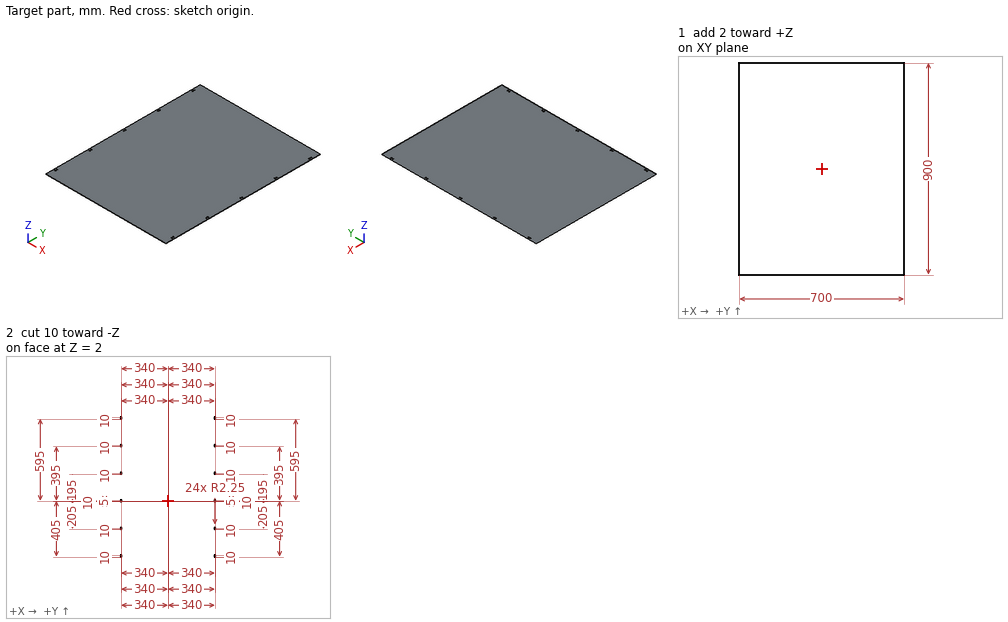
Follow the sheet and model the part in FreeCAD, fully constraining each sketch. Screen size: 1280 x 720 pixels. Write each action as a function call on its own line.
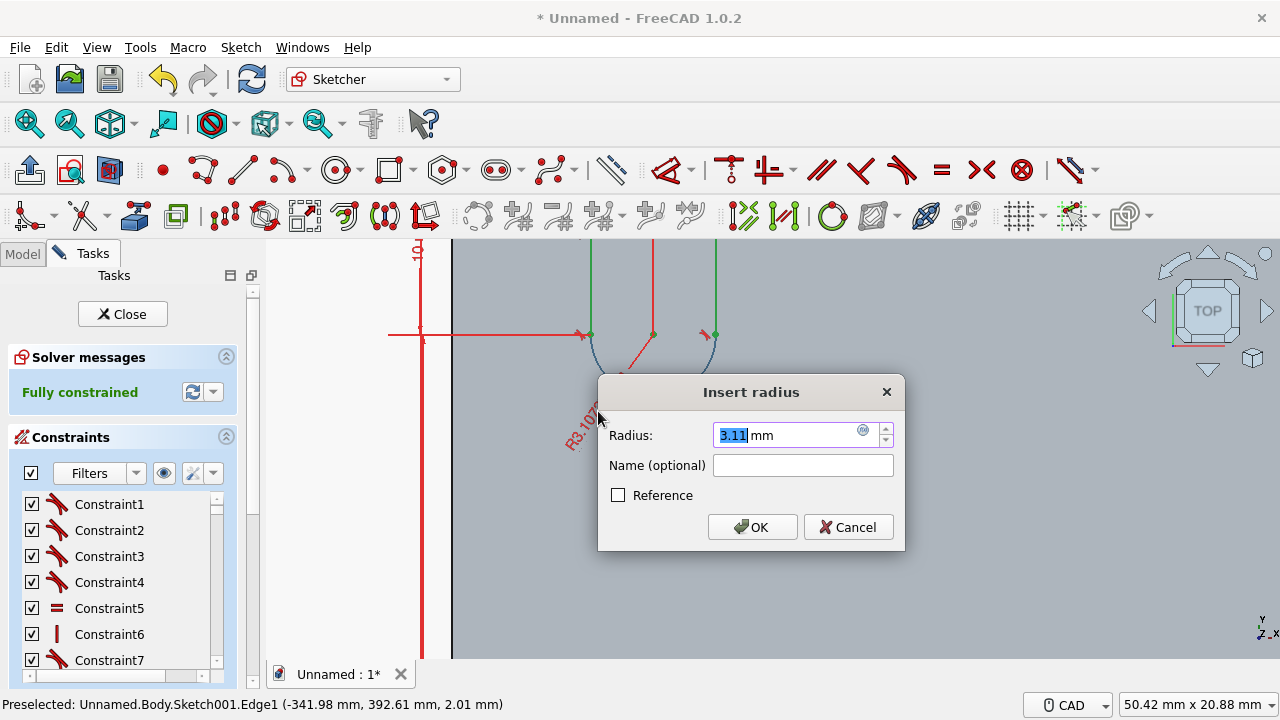
text(2.25)
key(Return)
key(Escape)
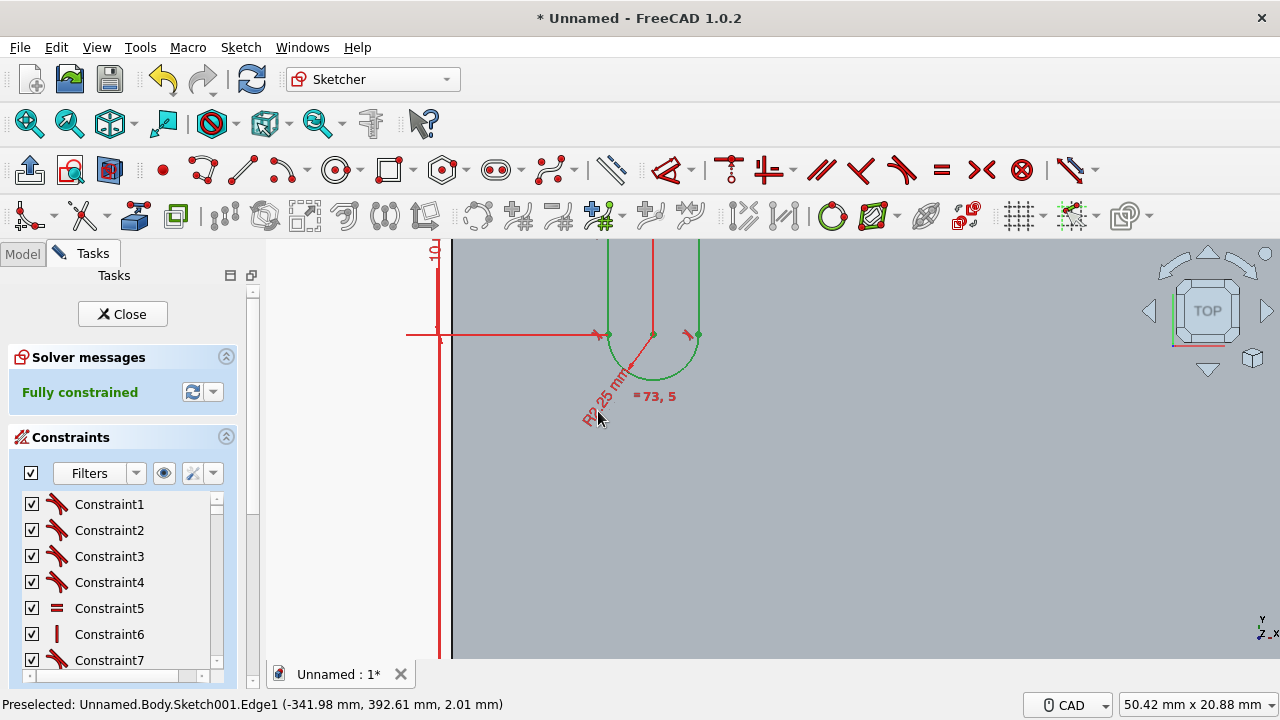
click(123, 314)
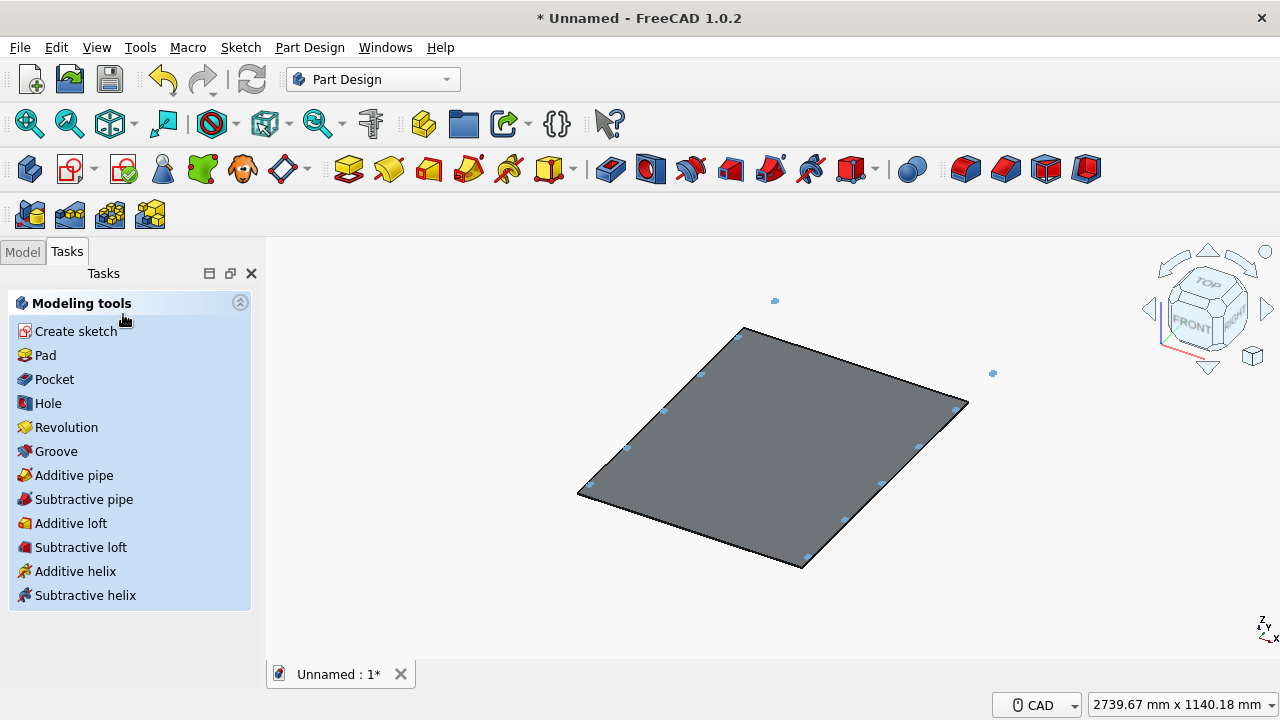
click(612, 170)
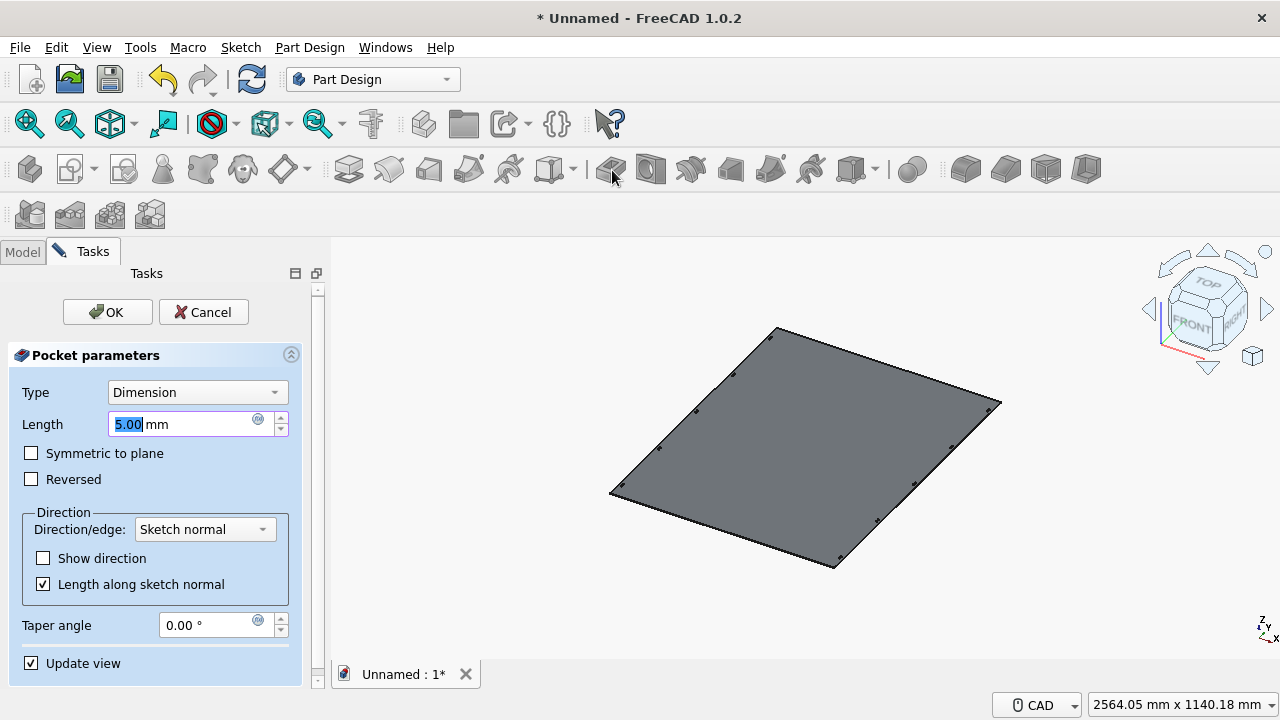
text(10)
key(Tab)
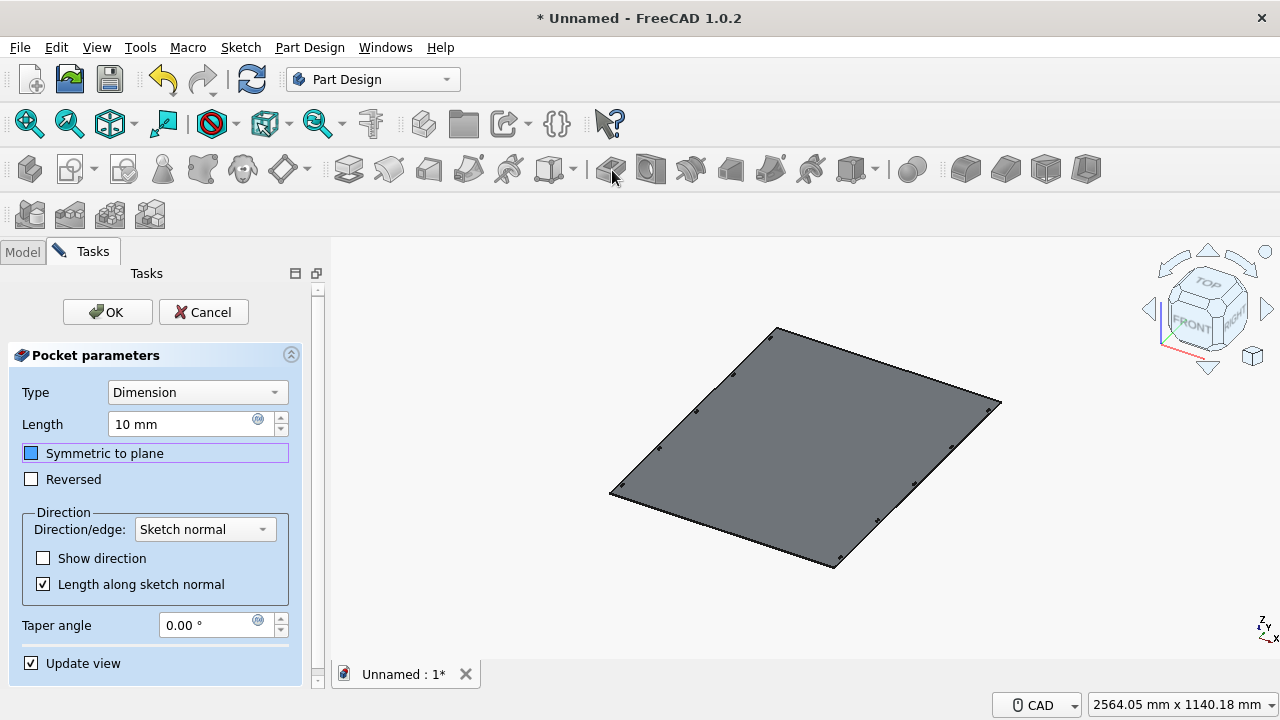
click(108, 312)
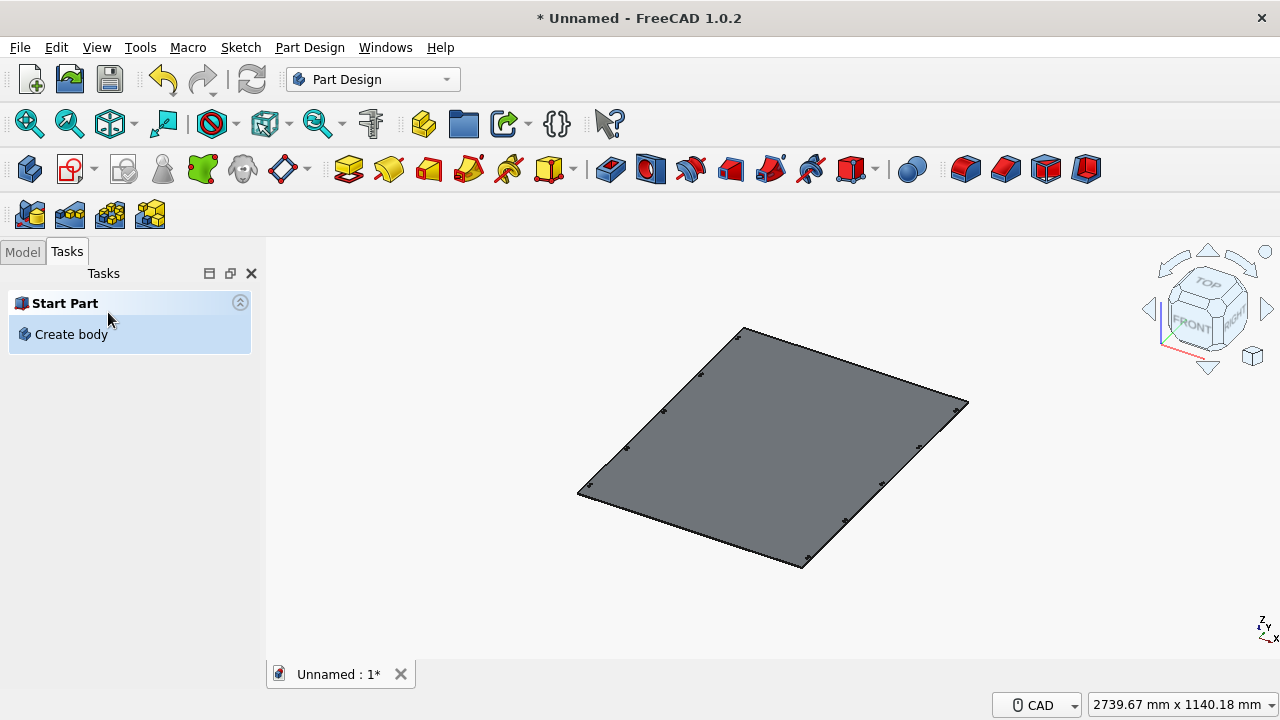
key(0)